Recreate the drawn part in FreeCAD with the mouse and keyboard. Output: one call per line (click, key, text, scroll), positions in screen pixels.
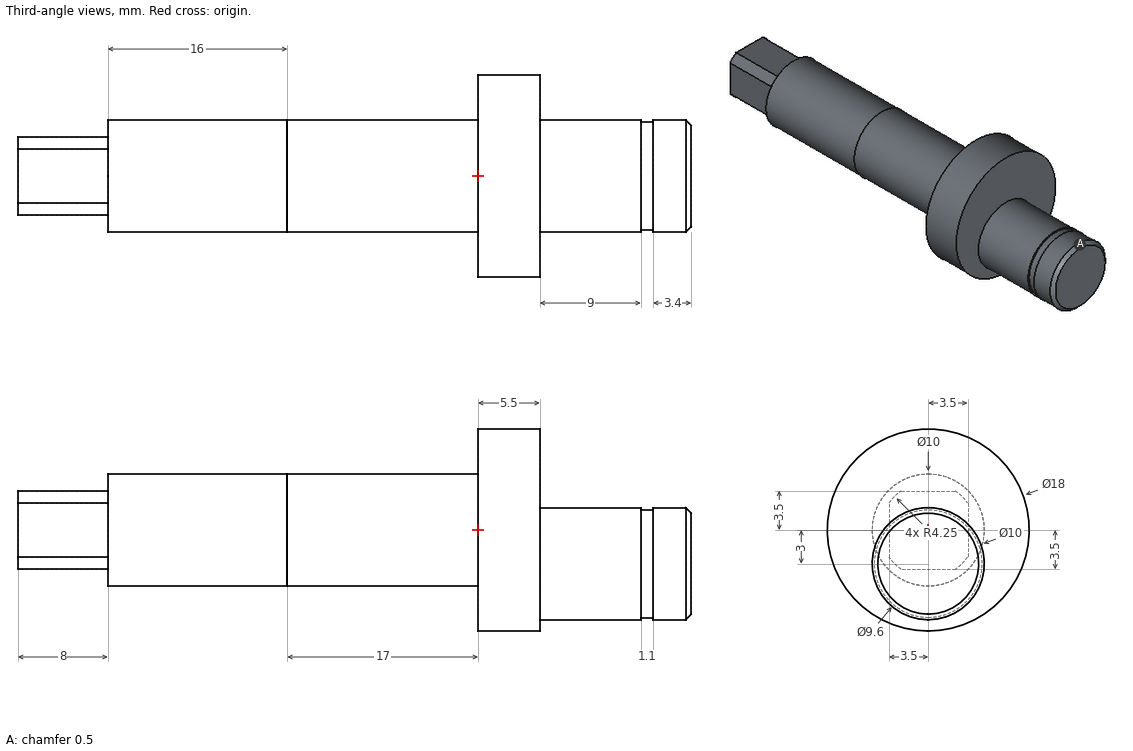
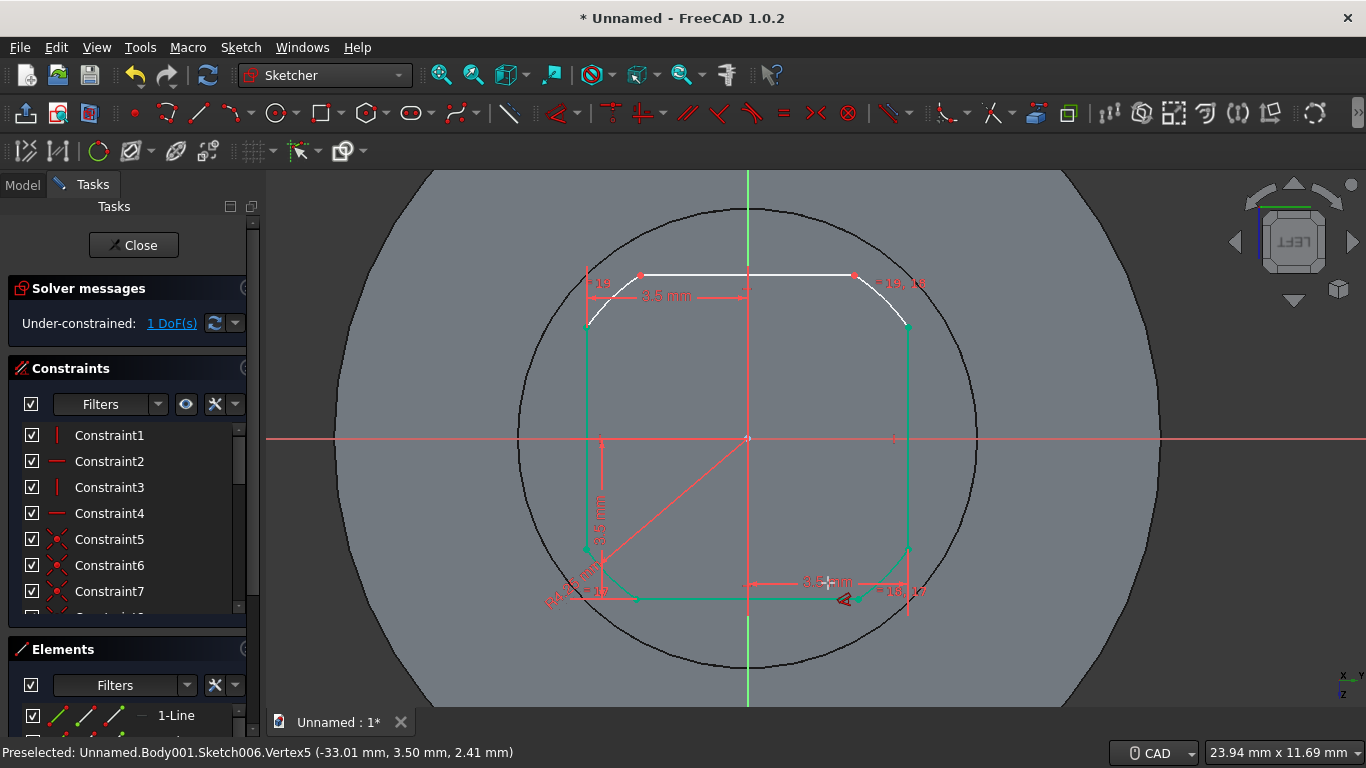
click(855, 275)
click(889, 357)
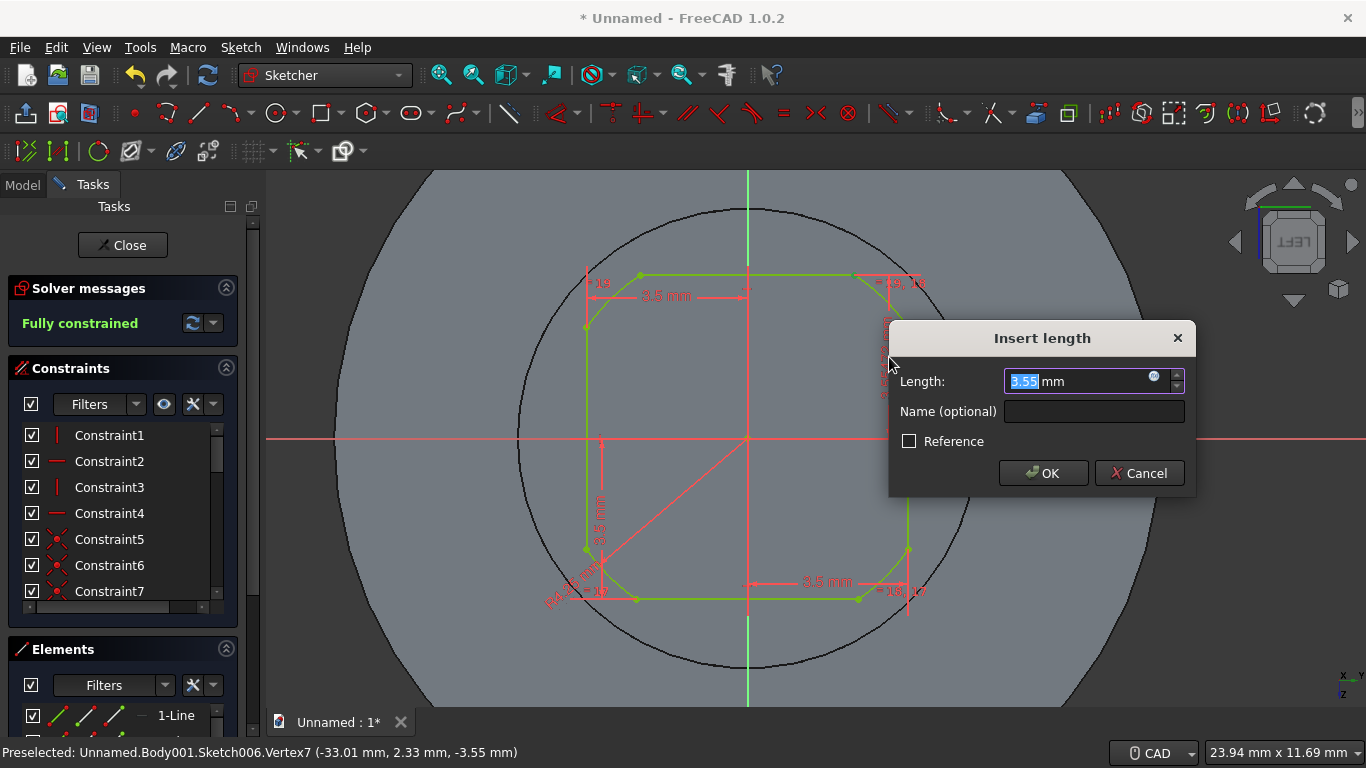
text(3.5)
key(Return)
key(Escape)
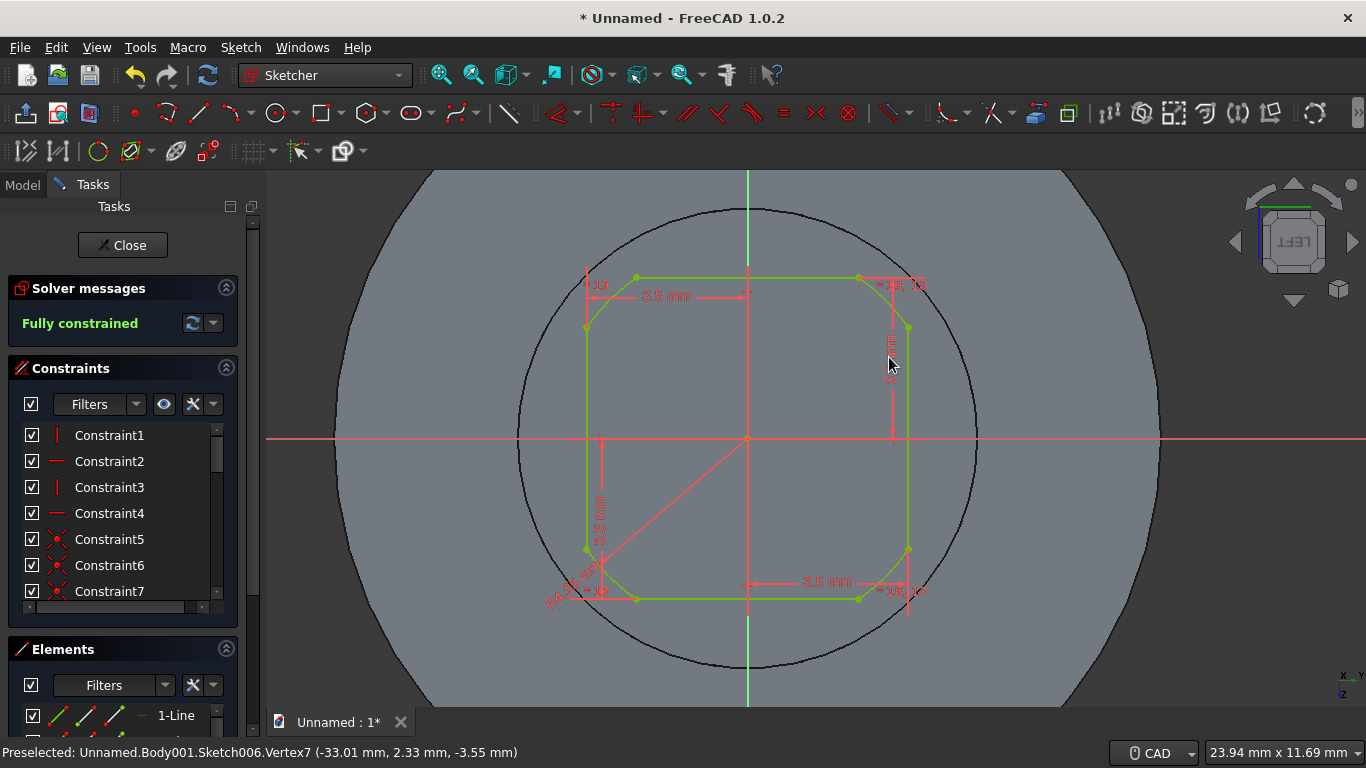
click(123, 245)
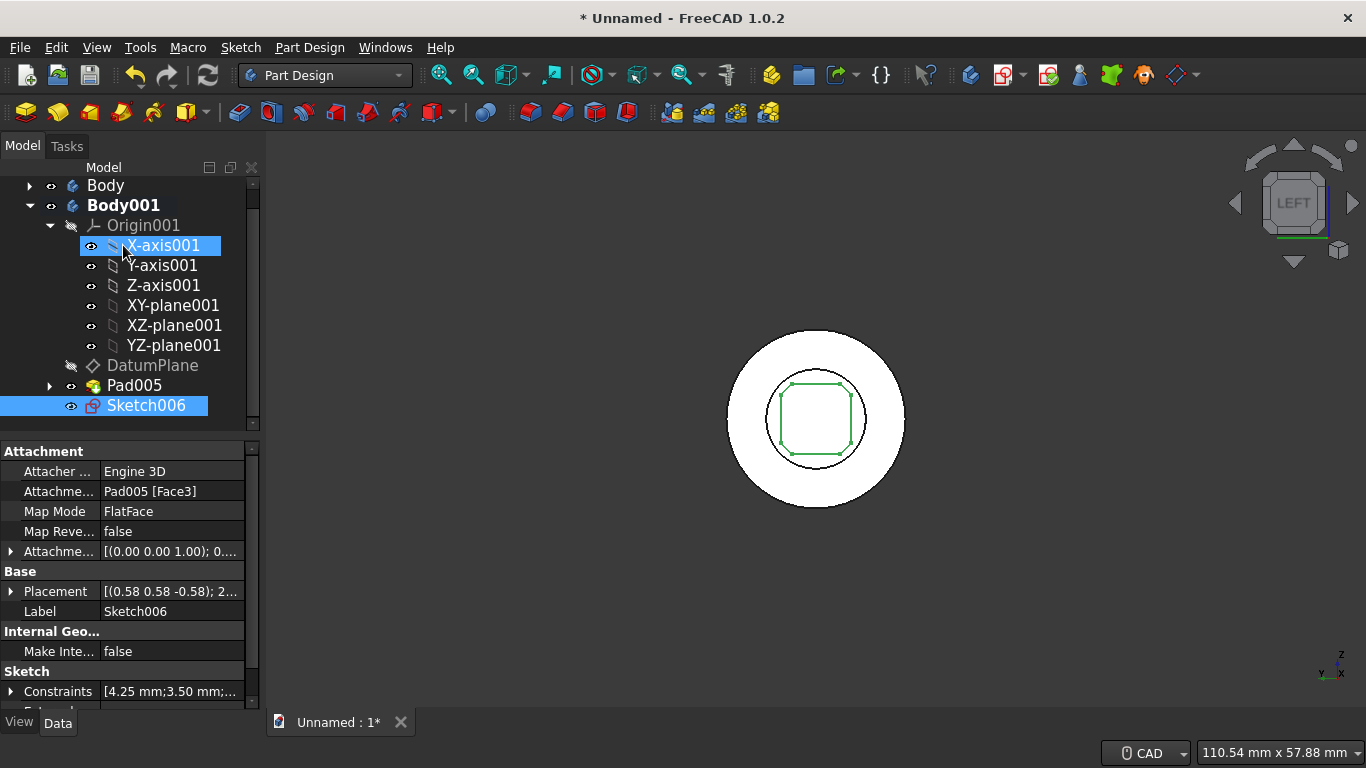
click(26, 112)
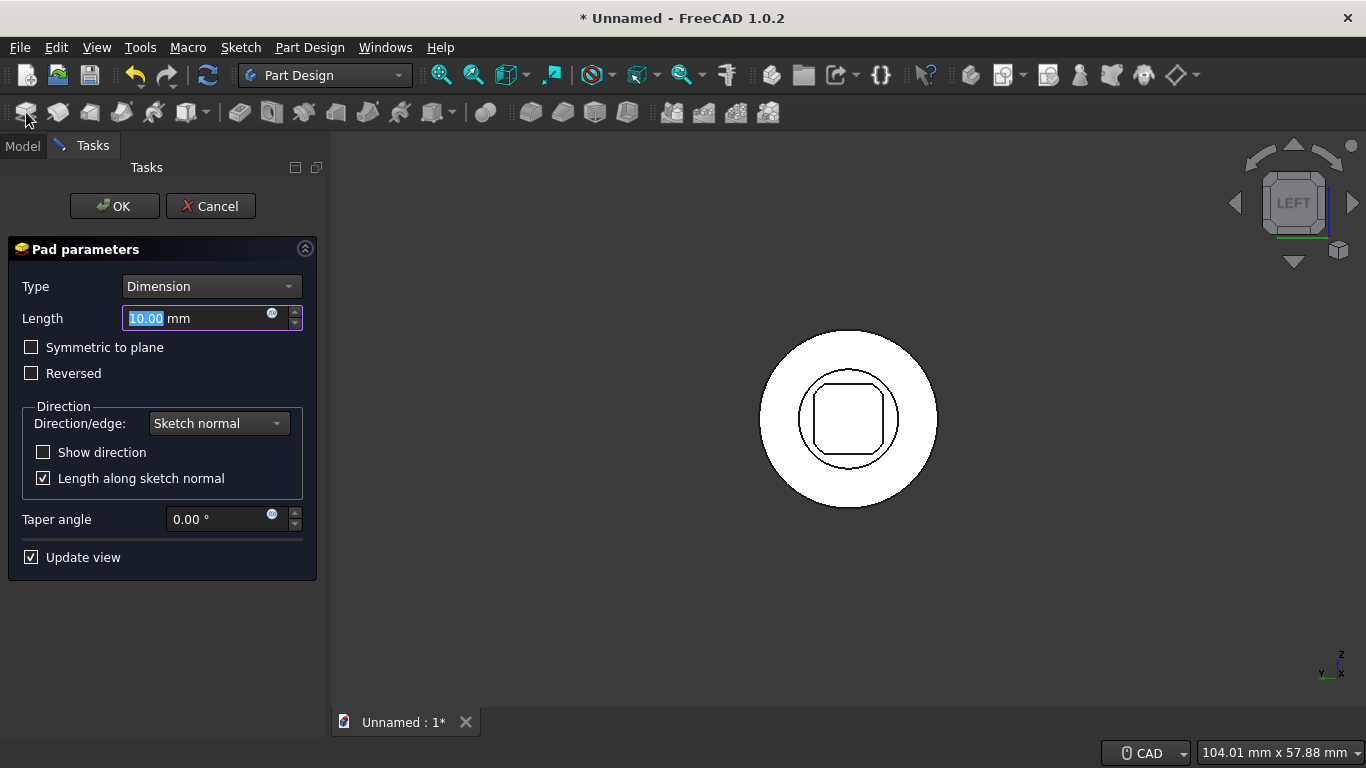
text(8)
key(Tab)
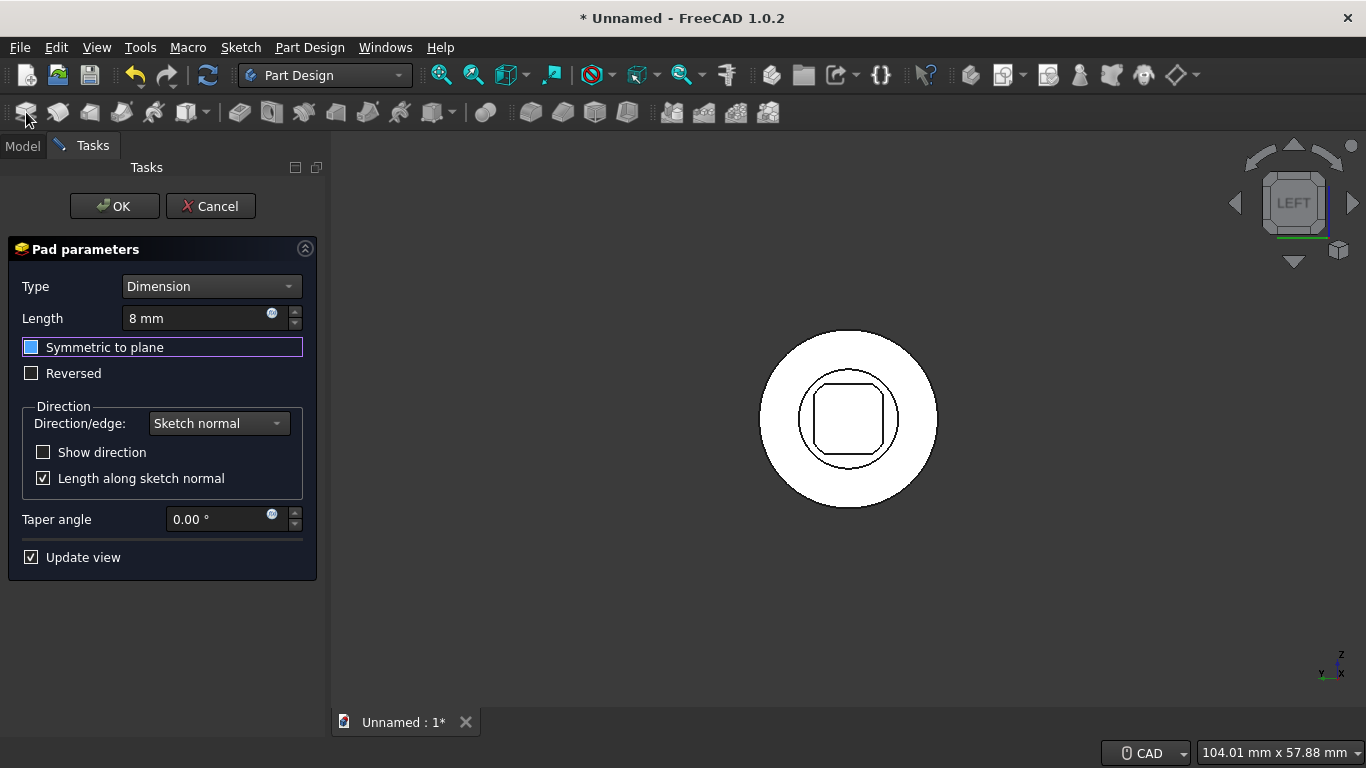
click(115, 206)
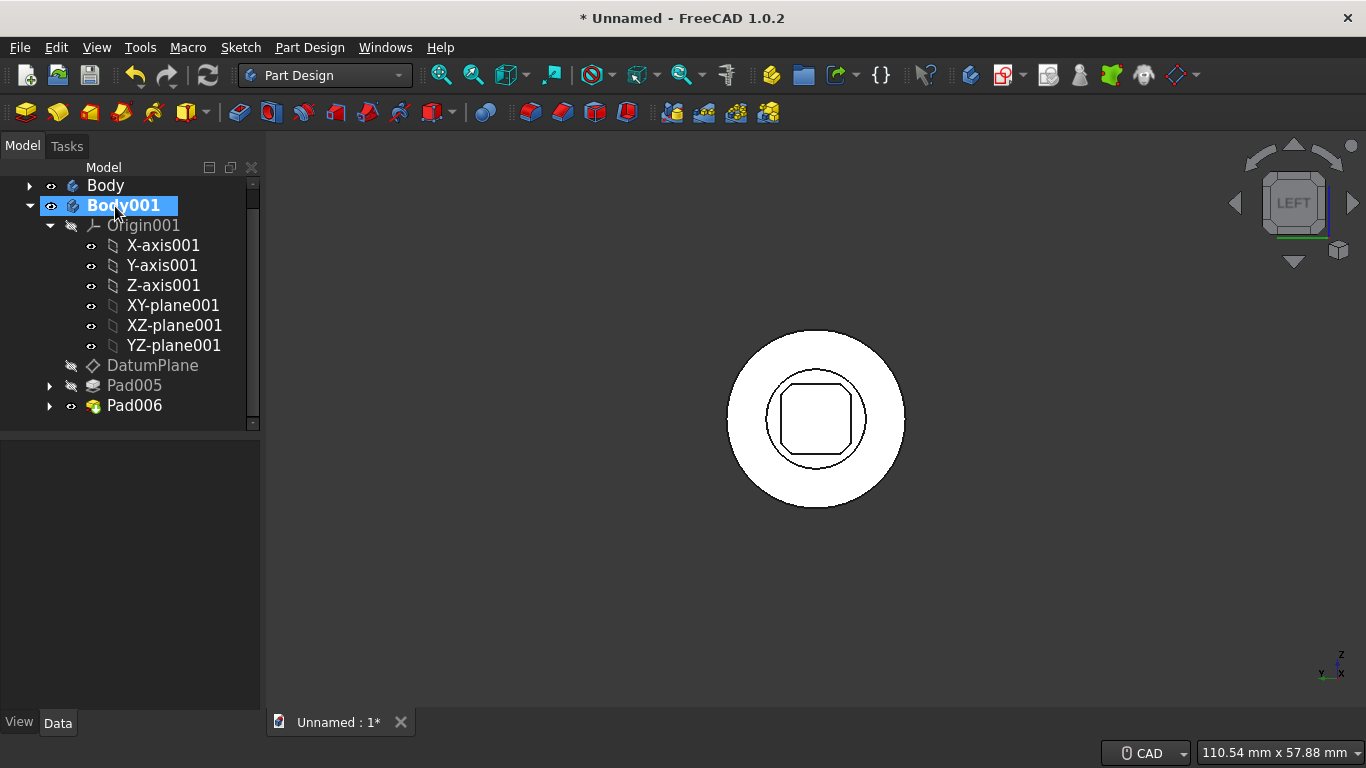
key(0)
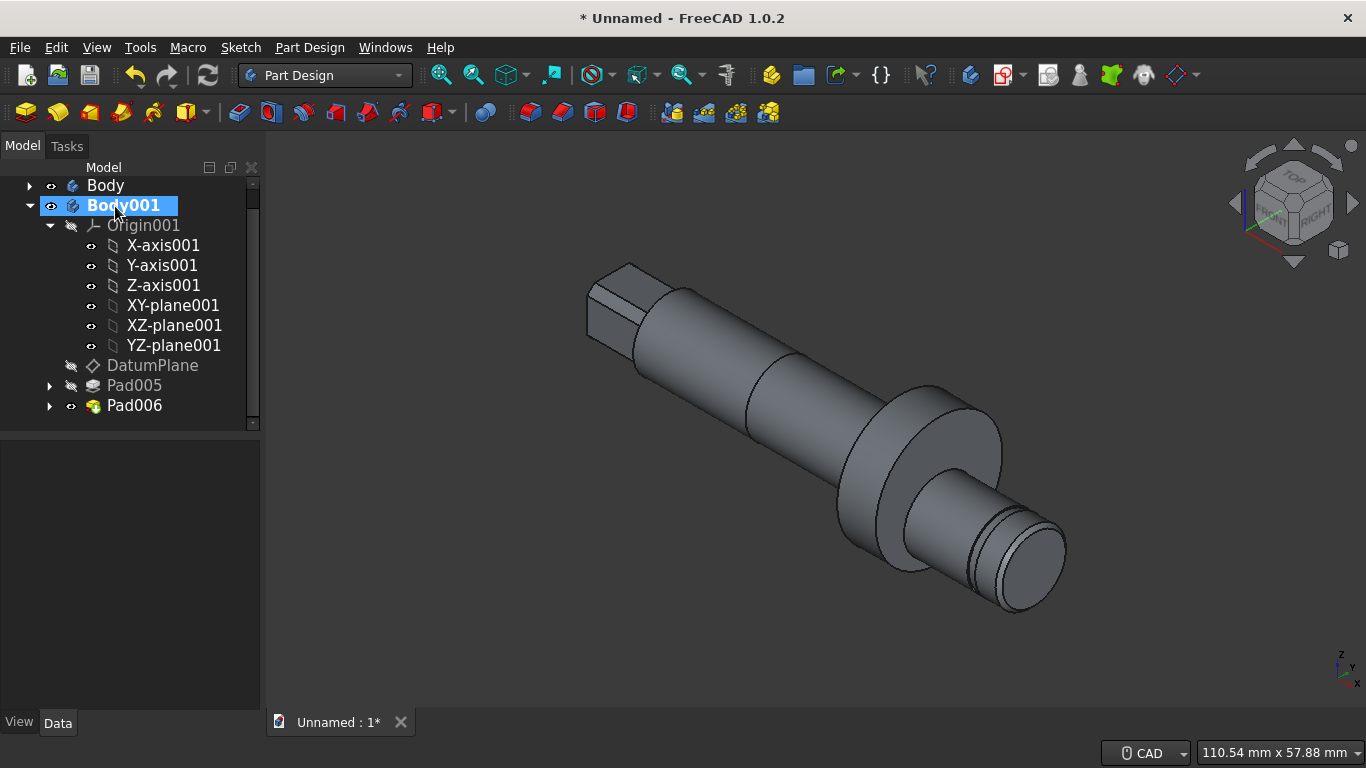
click(442, 76)